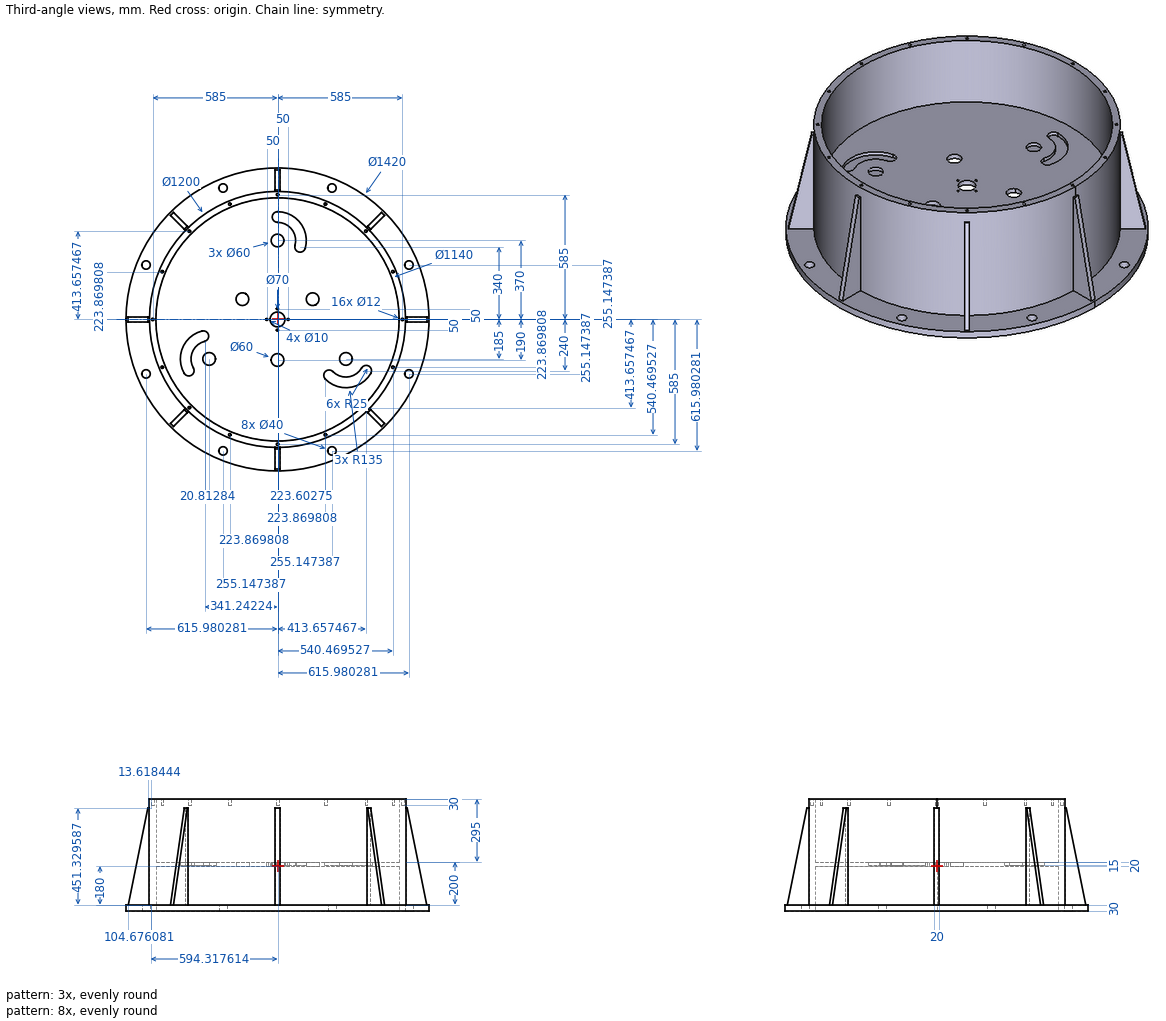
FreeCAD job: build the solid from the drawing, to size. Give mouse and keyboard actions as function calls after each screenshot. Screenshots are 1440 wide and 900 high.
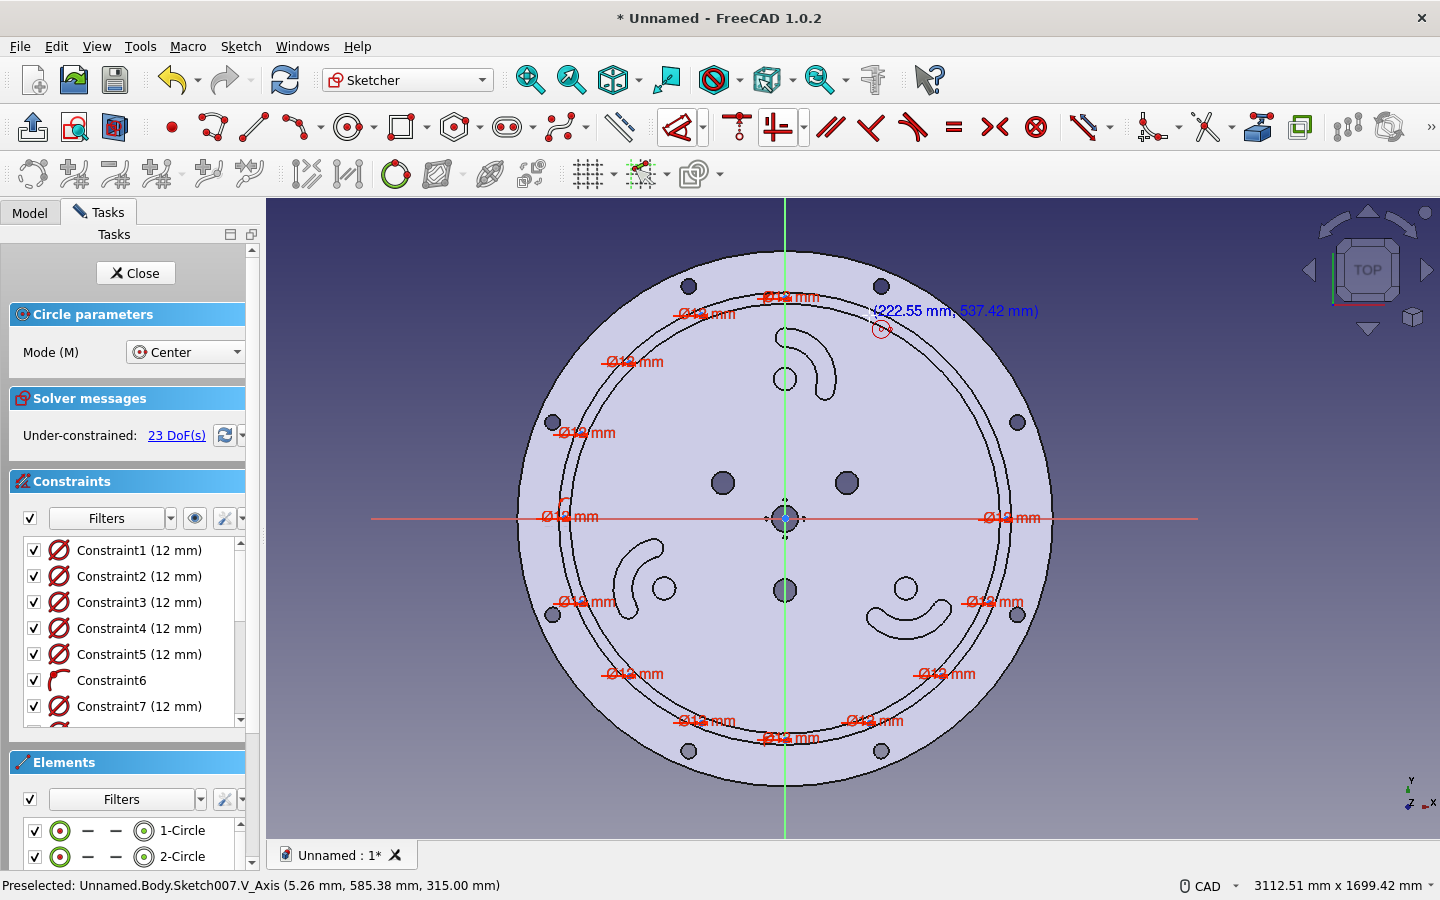
click(869, 315)
move(871, 313)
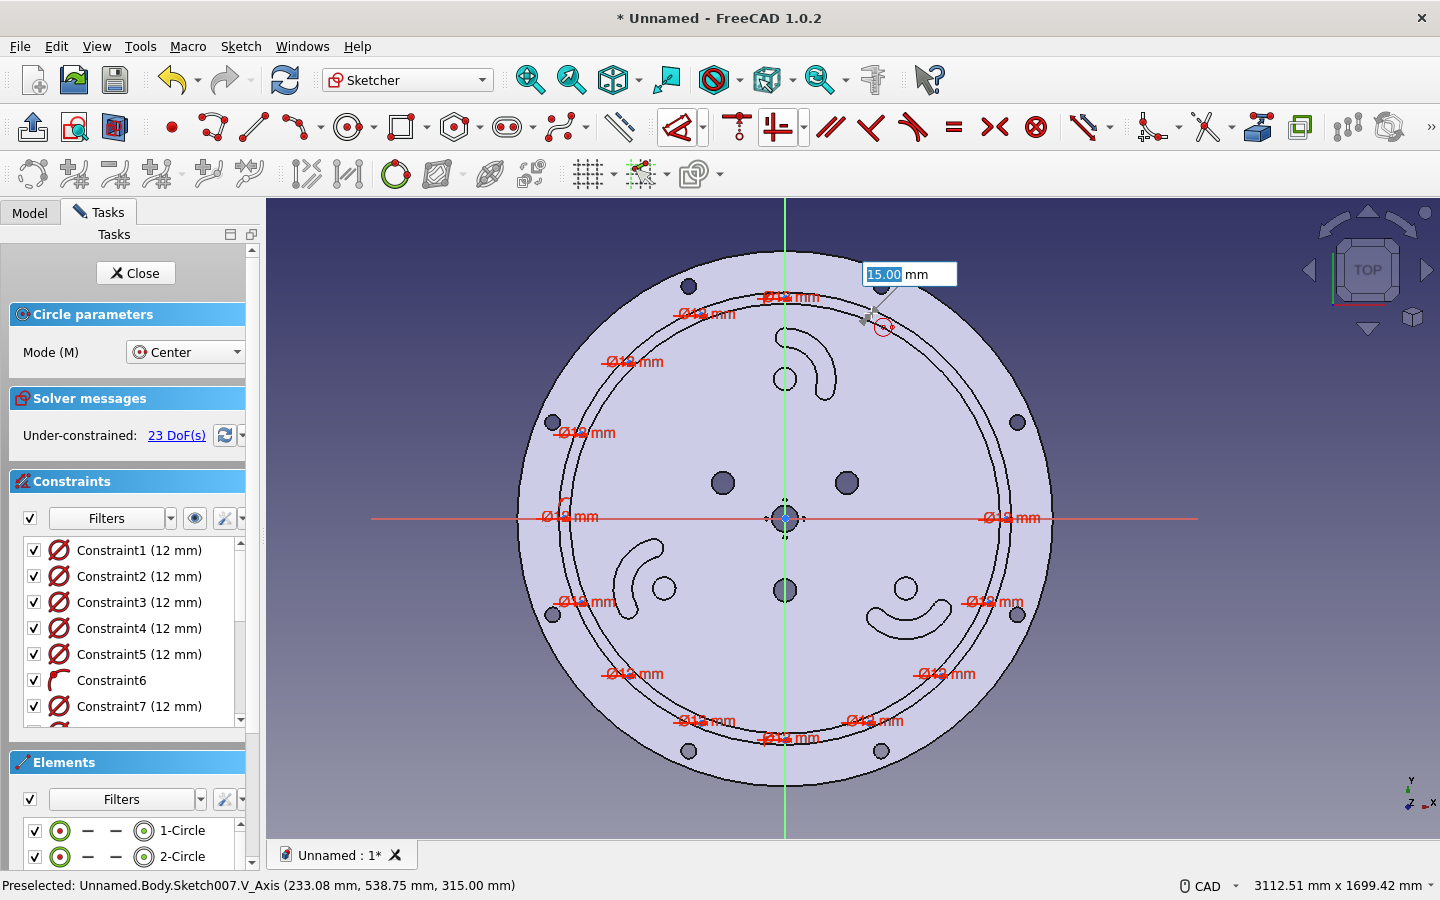
text(12)
key(Return)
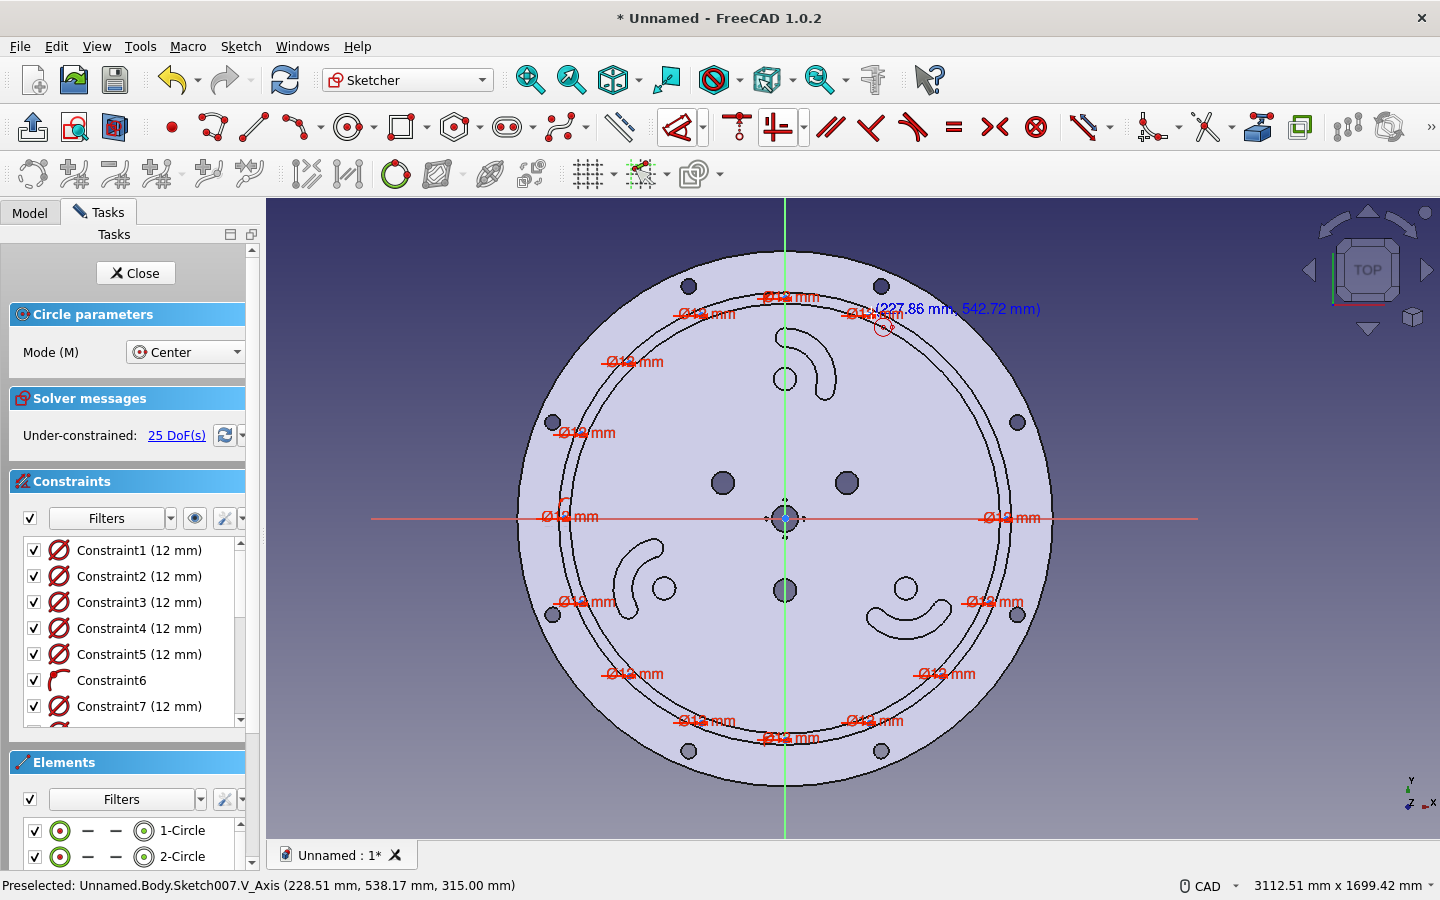
scroll(941, 363, up, 12)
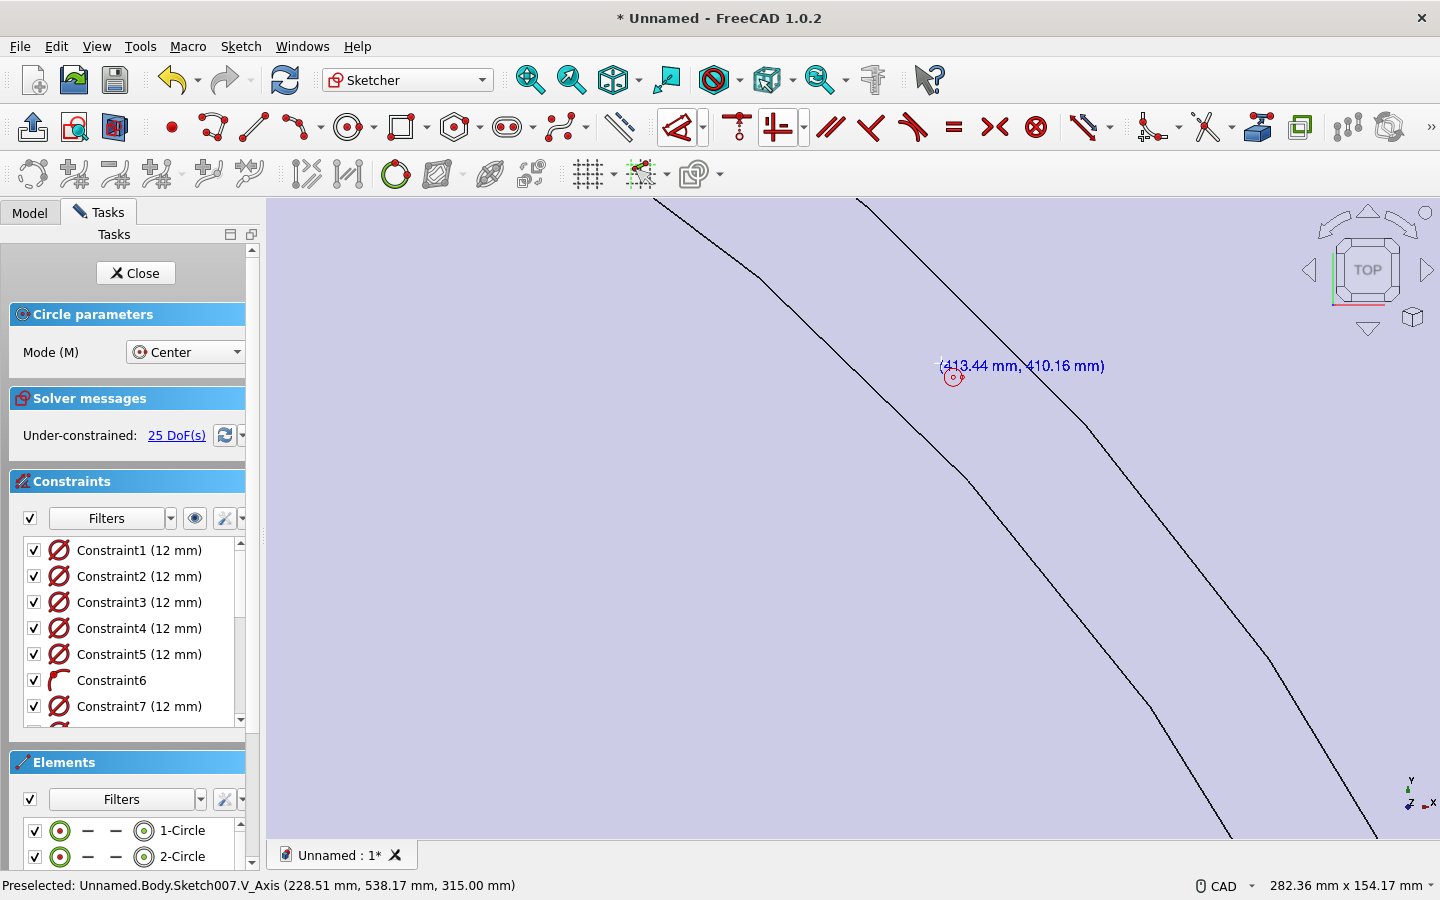
scroll(941, 363, down, 12)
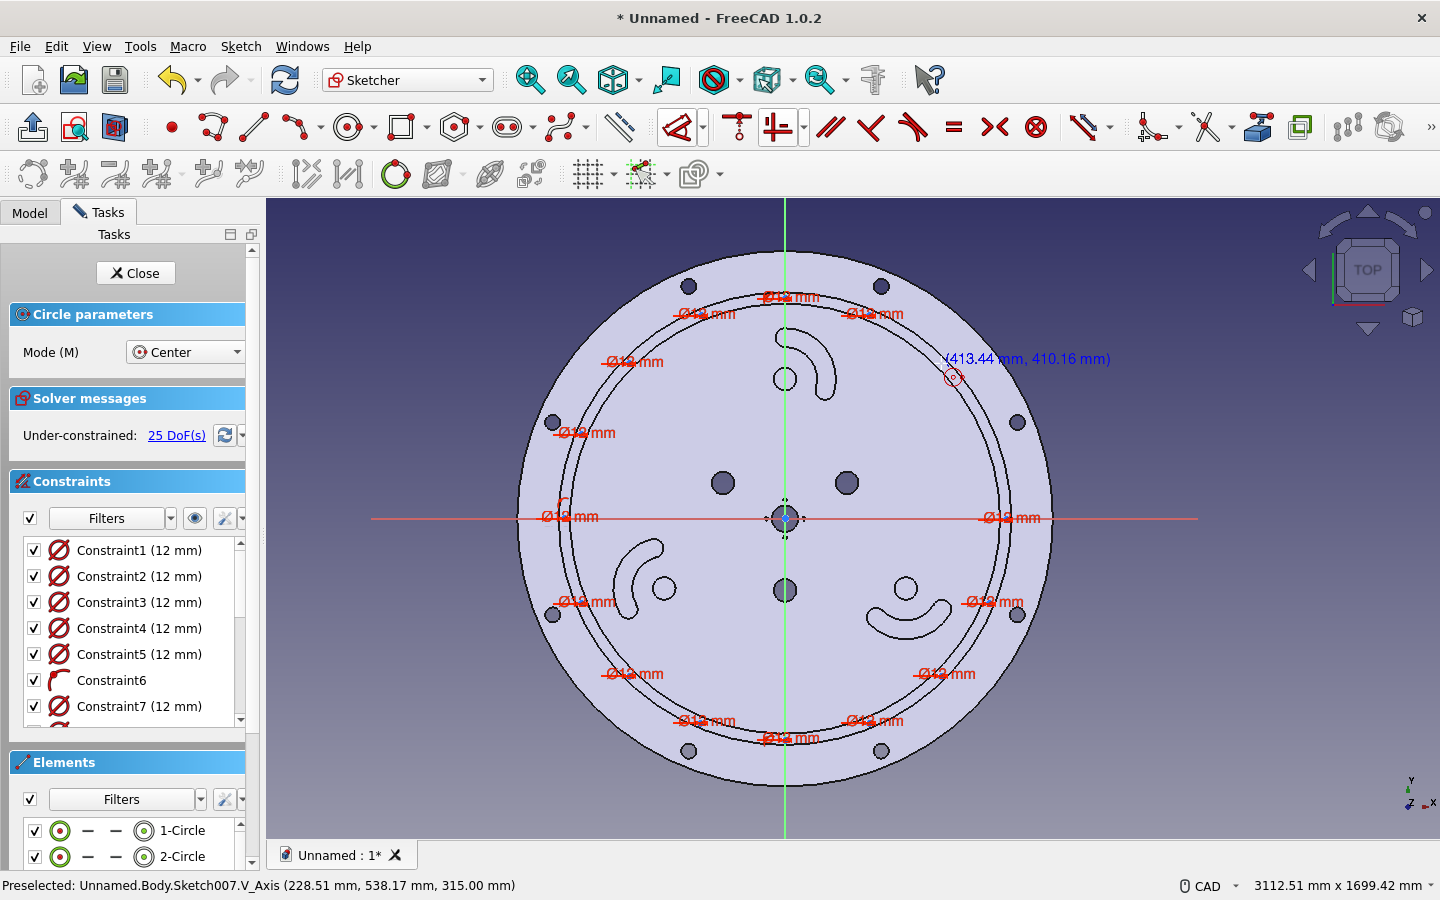
click(941, 363)
move(943, 361)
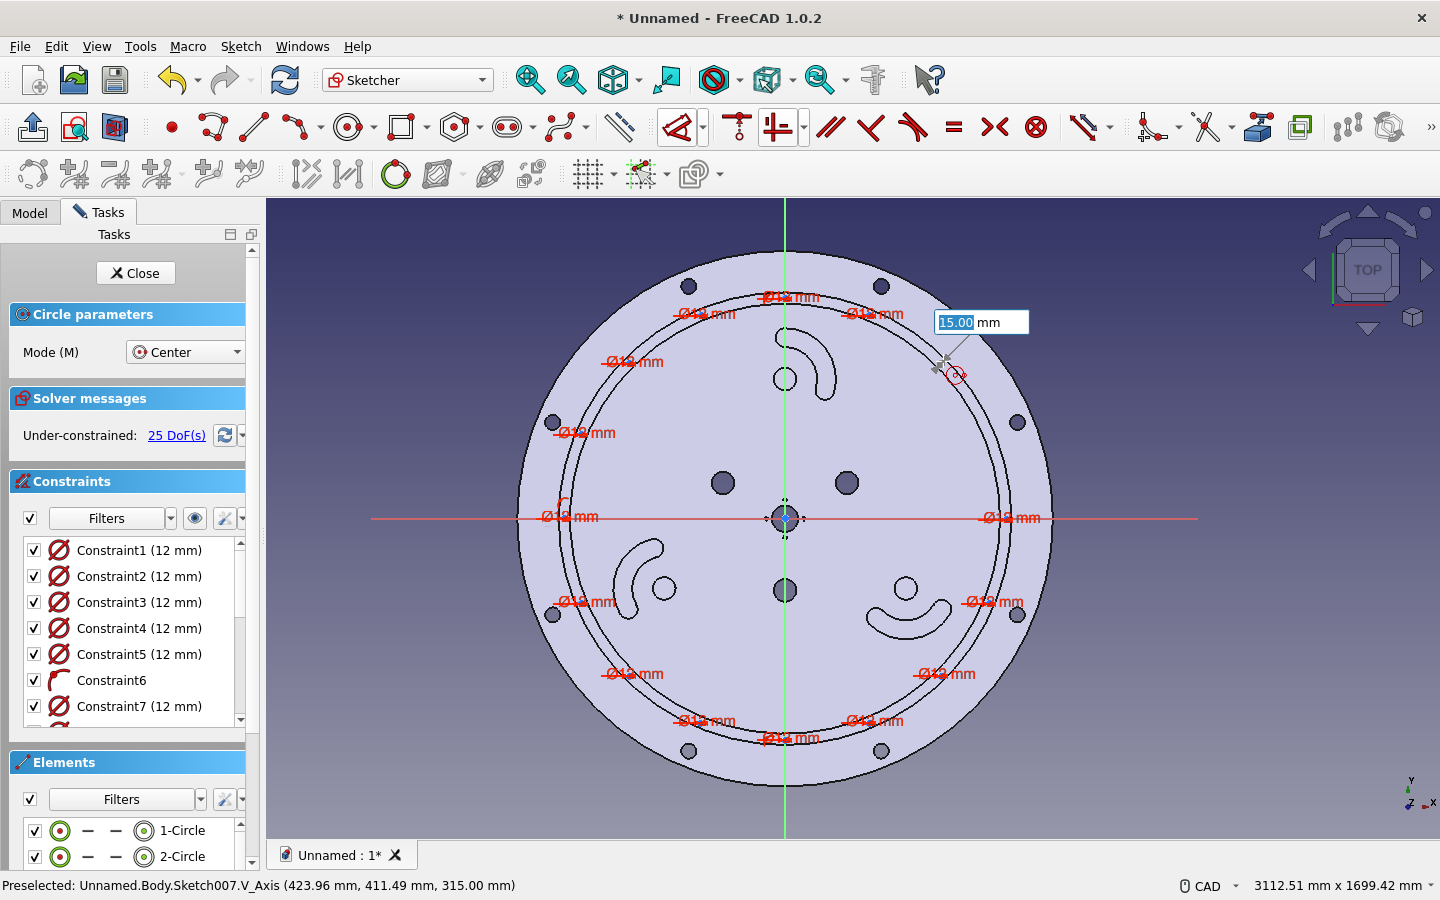
text(12)
key(Return)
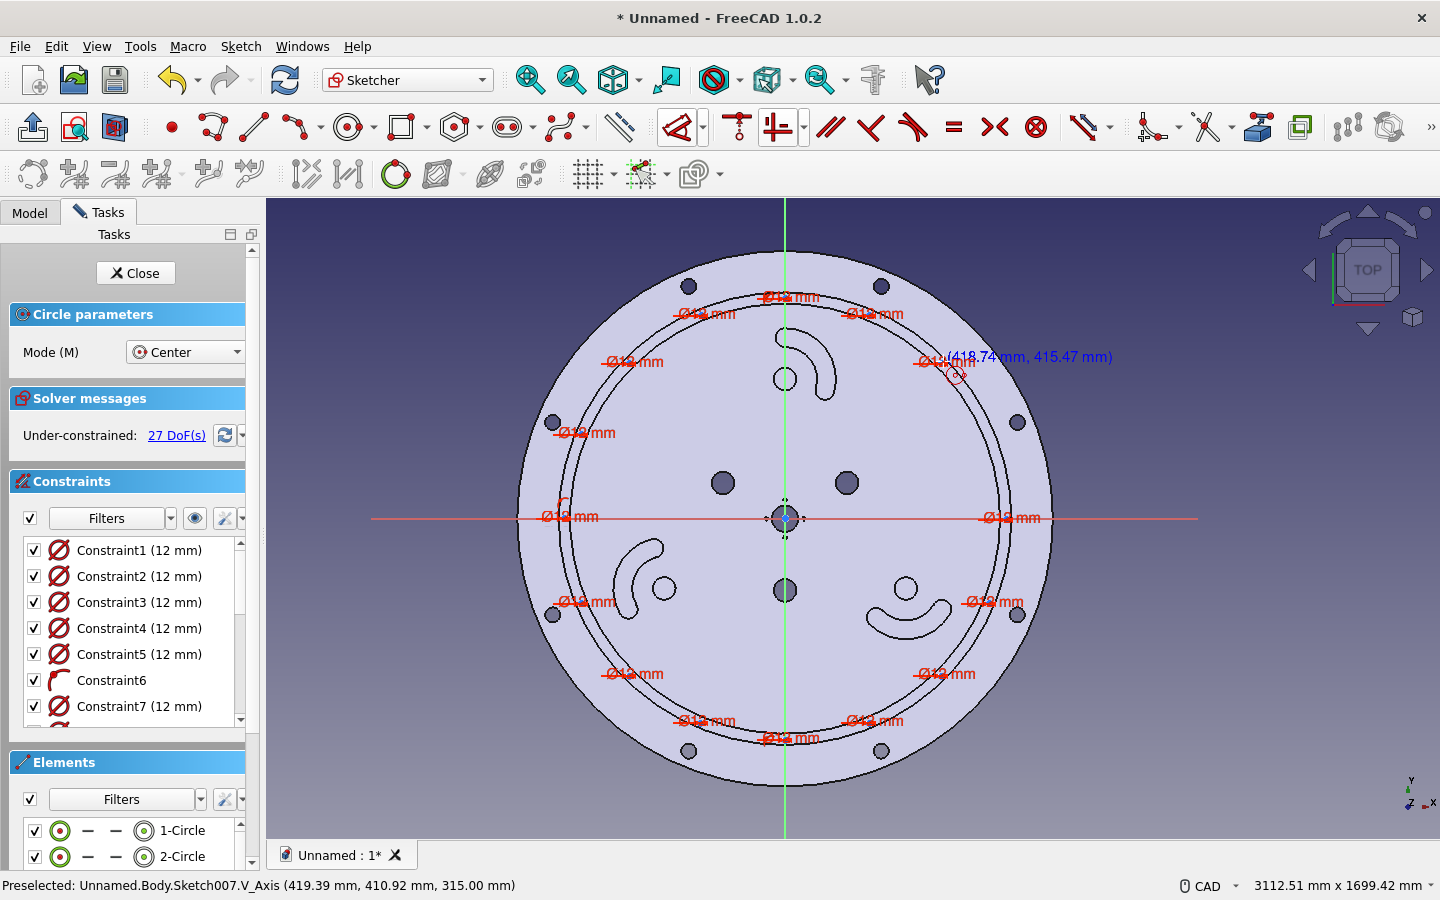
scroll(989, 434, up, 12)